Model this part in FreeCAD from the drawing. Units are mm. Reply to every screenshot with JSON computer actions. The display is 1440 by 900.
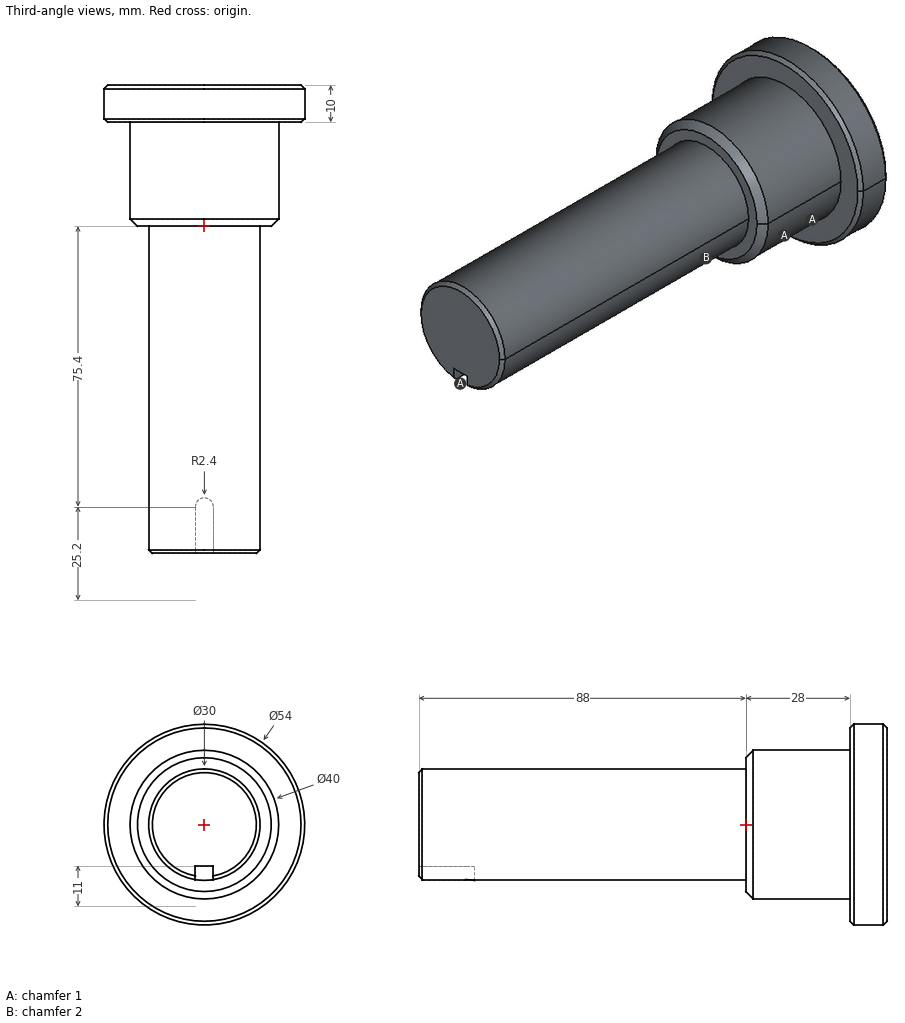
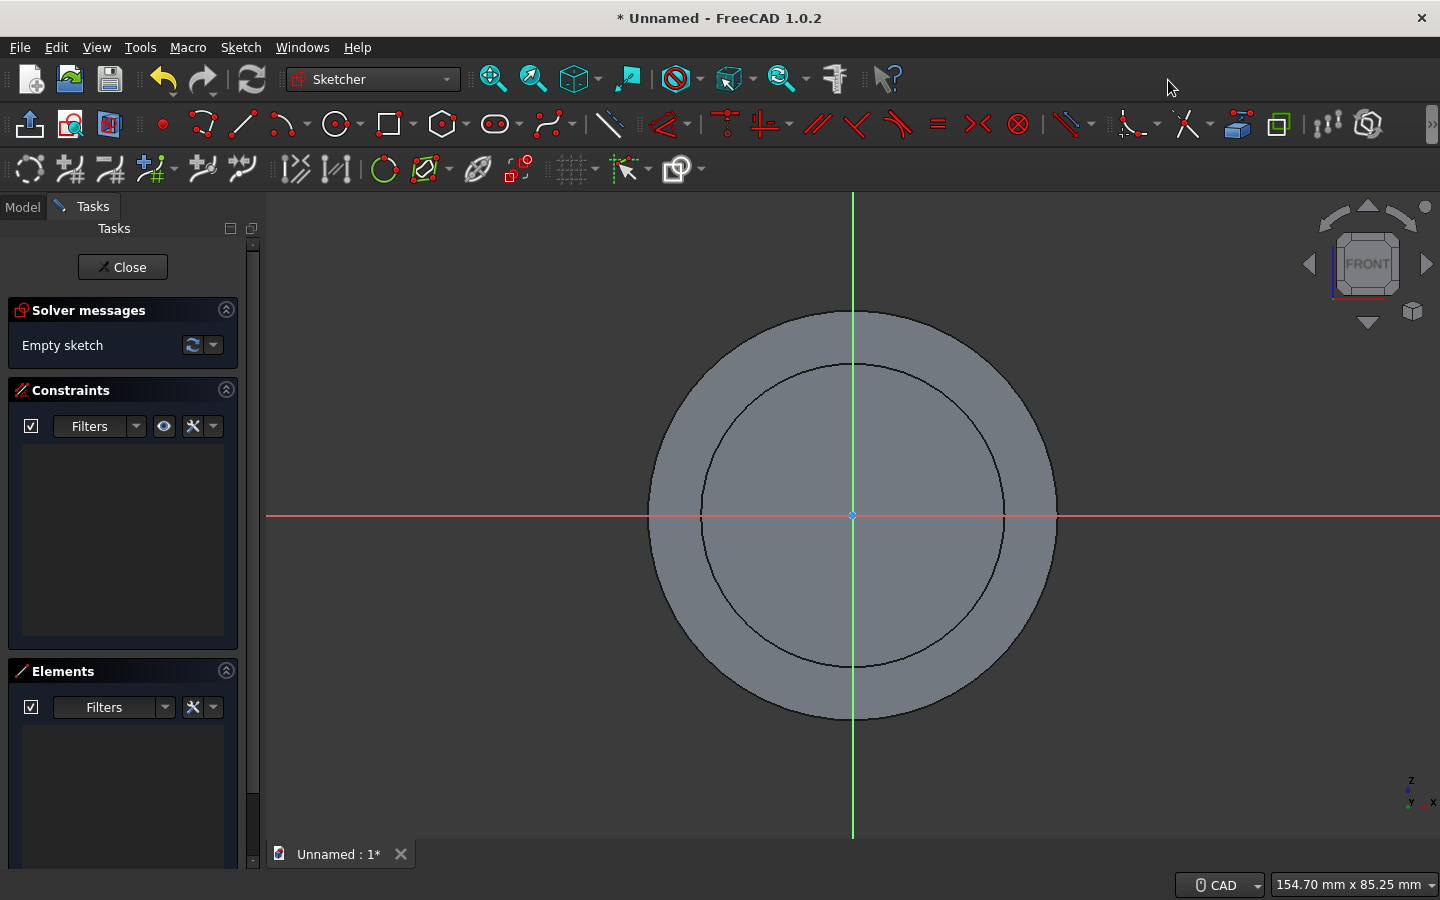
{"action": "scroll", "coordinate": [936, 516], "scroll_direction": "up", "scroll_amount": 3}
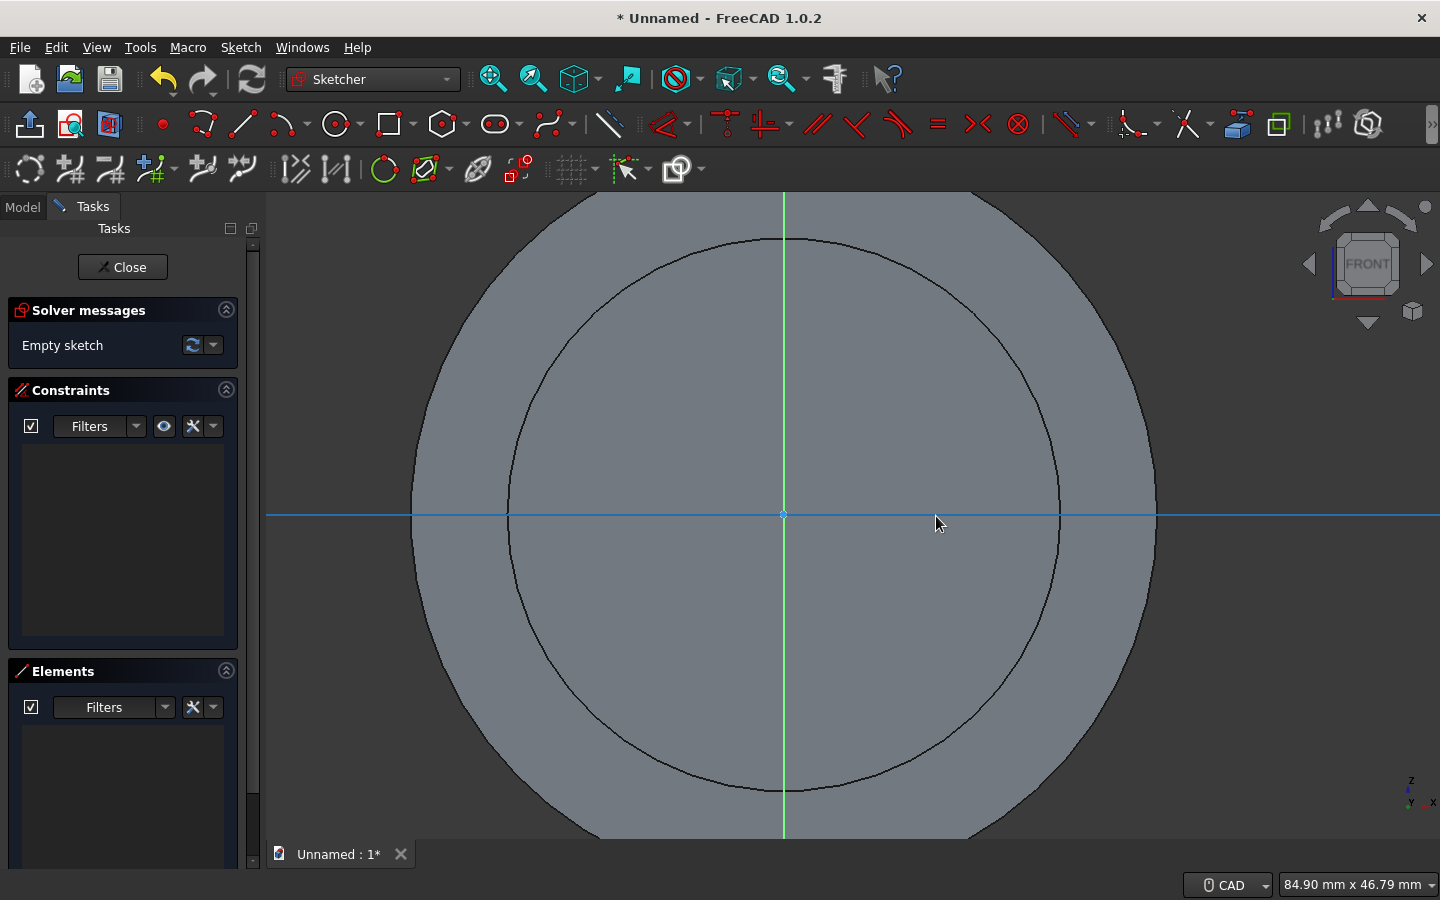
{"action": "left_click", "coordinate": [336, 124]}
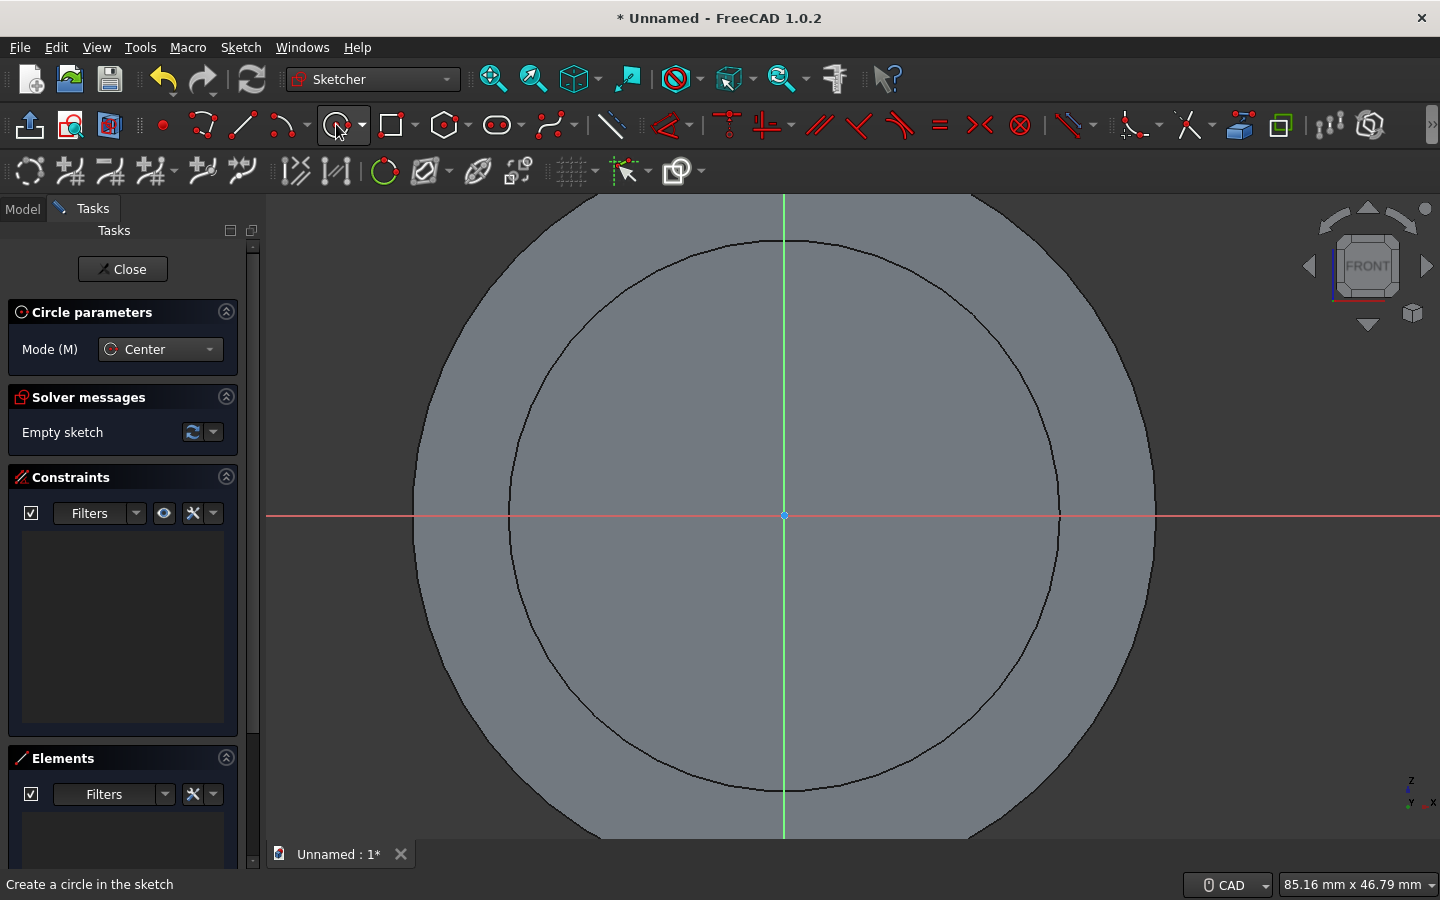
{"action": "left_click", "coordinate": [784, 516]}
{"action": "mouse_move", "coordinate": [930, 369]}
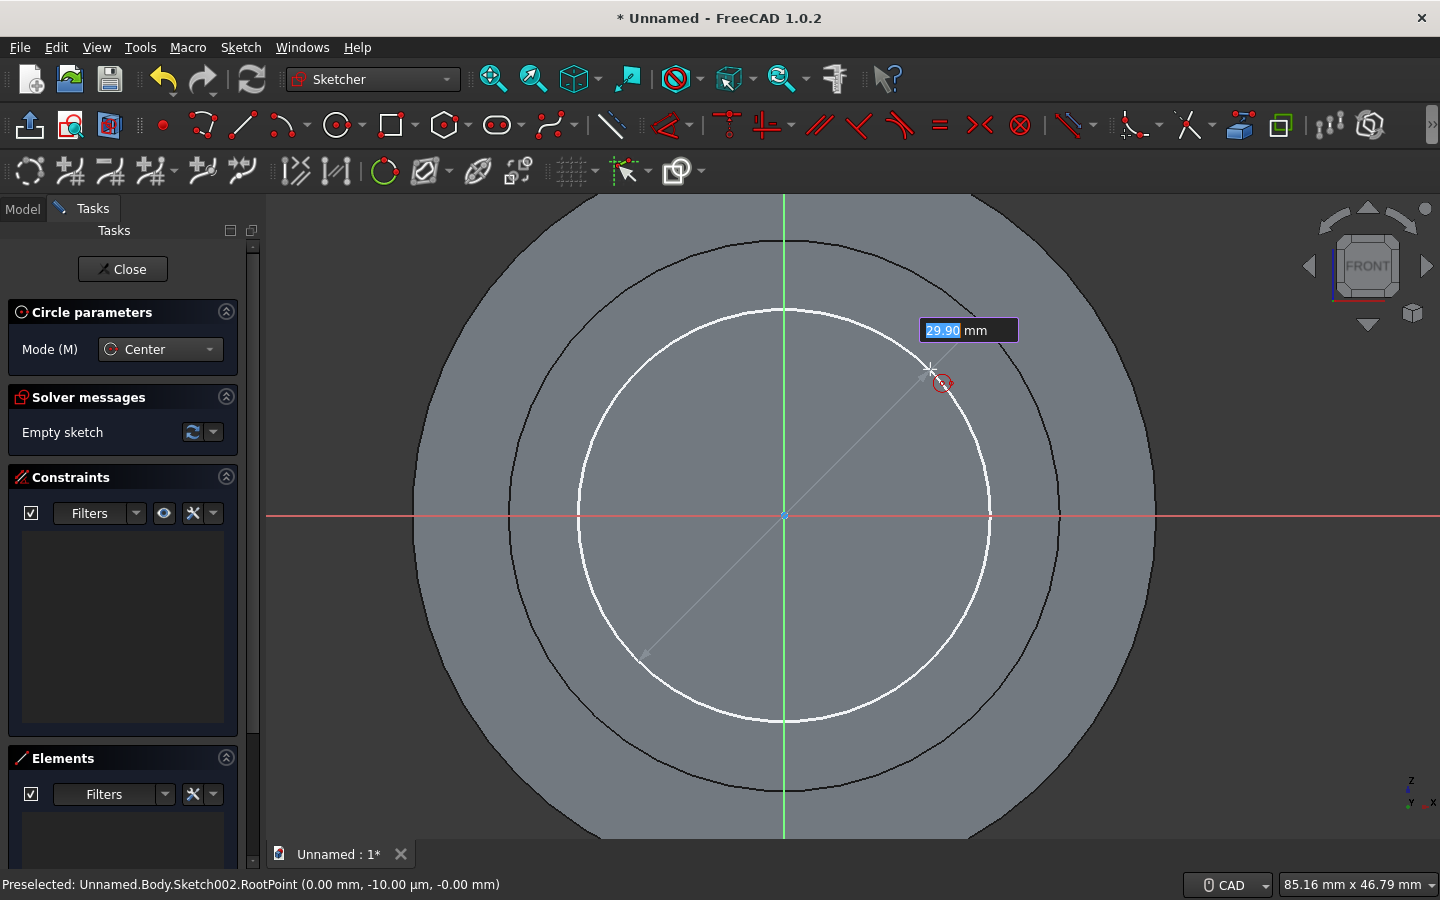
{"action": "type", "text": "30"}
{"action": "key", "text": "Return"}
{"action": "key", "text": "Escape"}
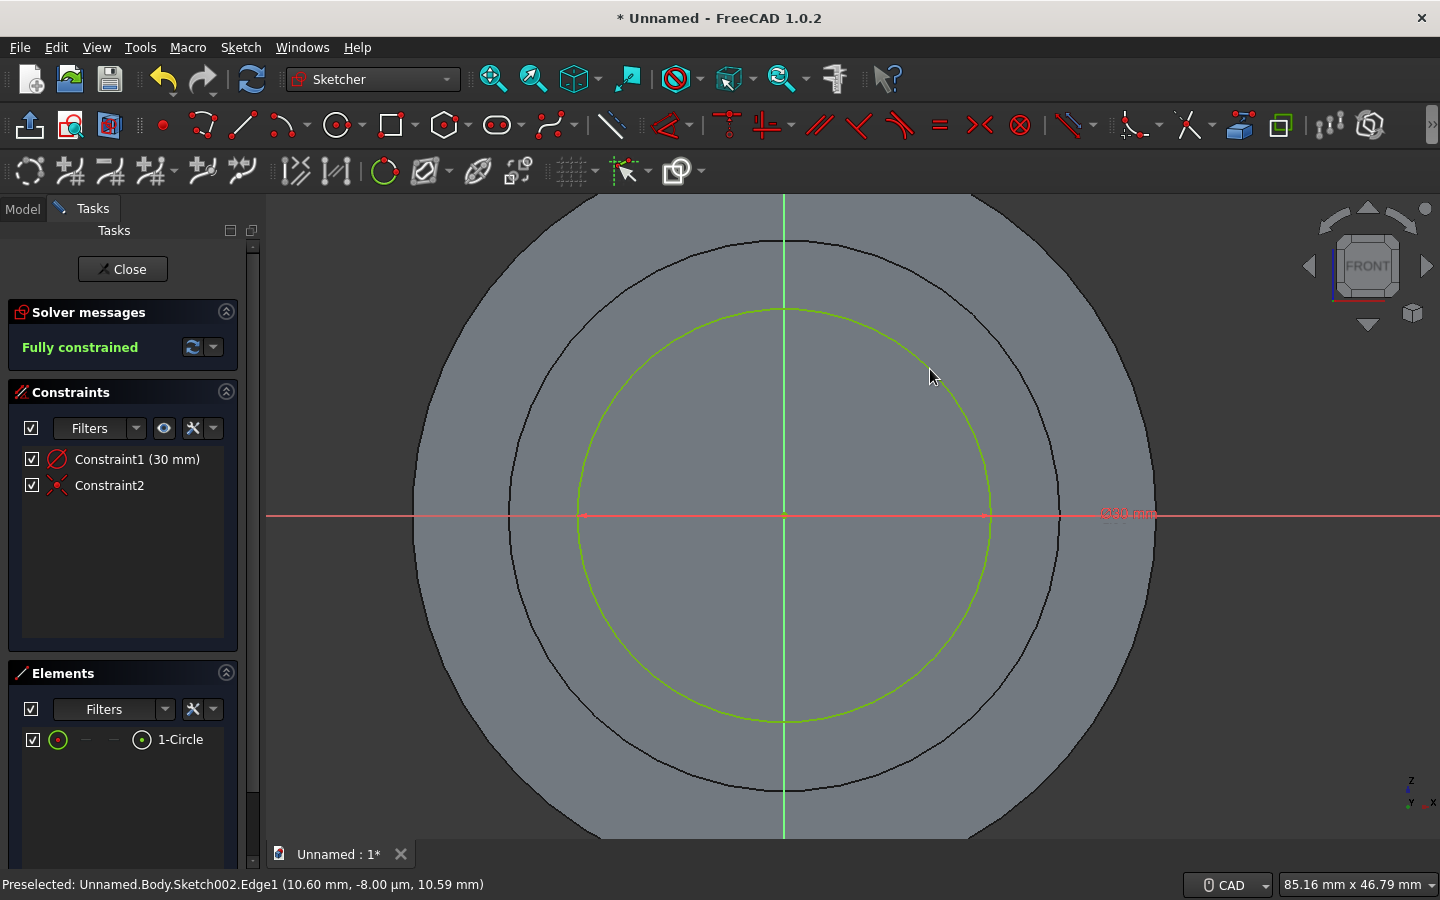
{"action": "left_click", "coordinate": [123, 269]}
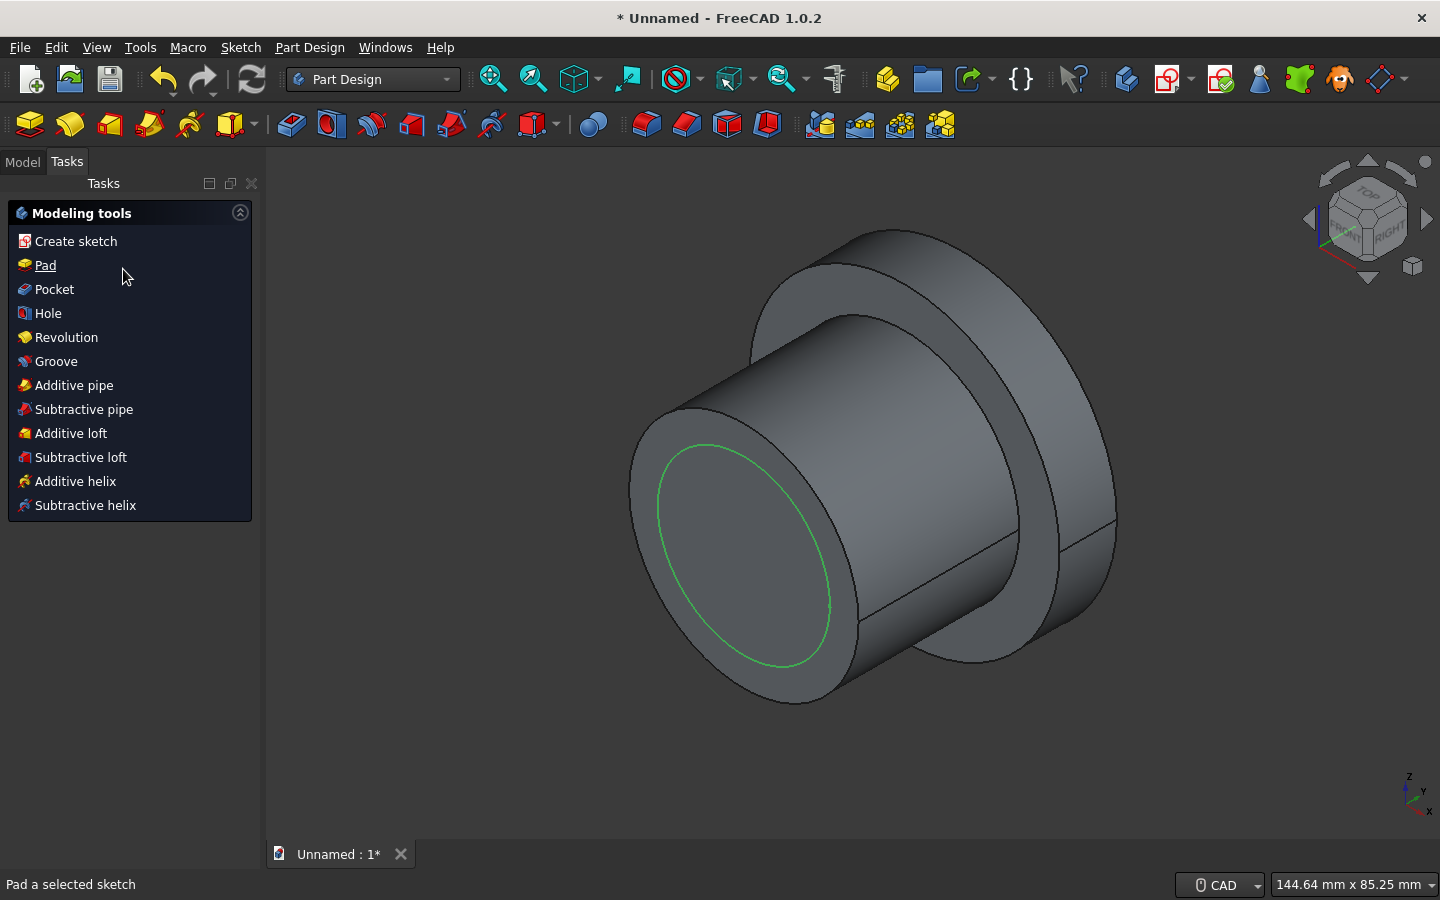
{"action": "left_click", "coordinate": [30, 124]}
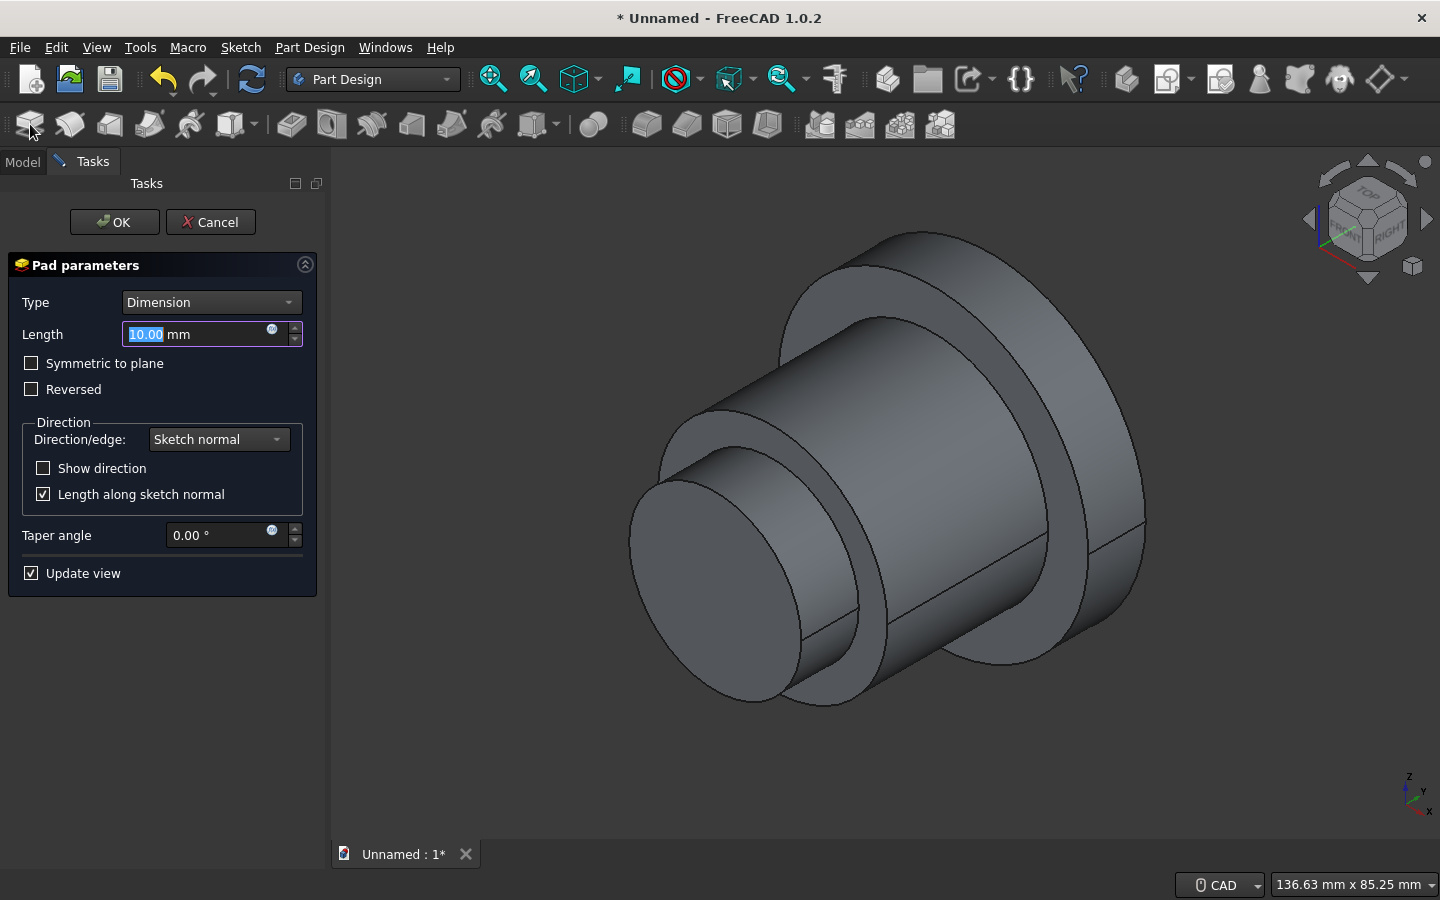
{"action": "type", "text": "88"}
{"action": "key", "text": "Tab"}